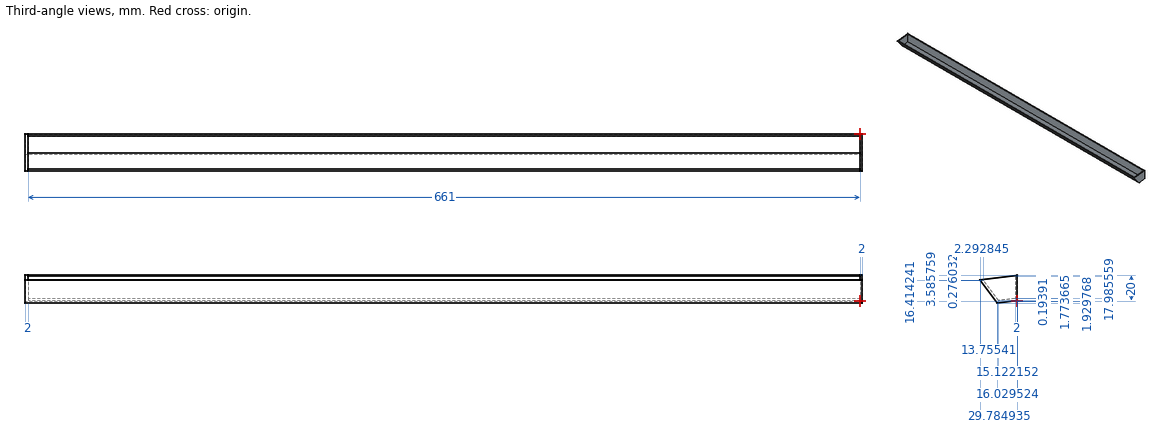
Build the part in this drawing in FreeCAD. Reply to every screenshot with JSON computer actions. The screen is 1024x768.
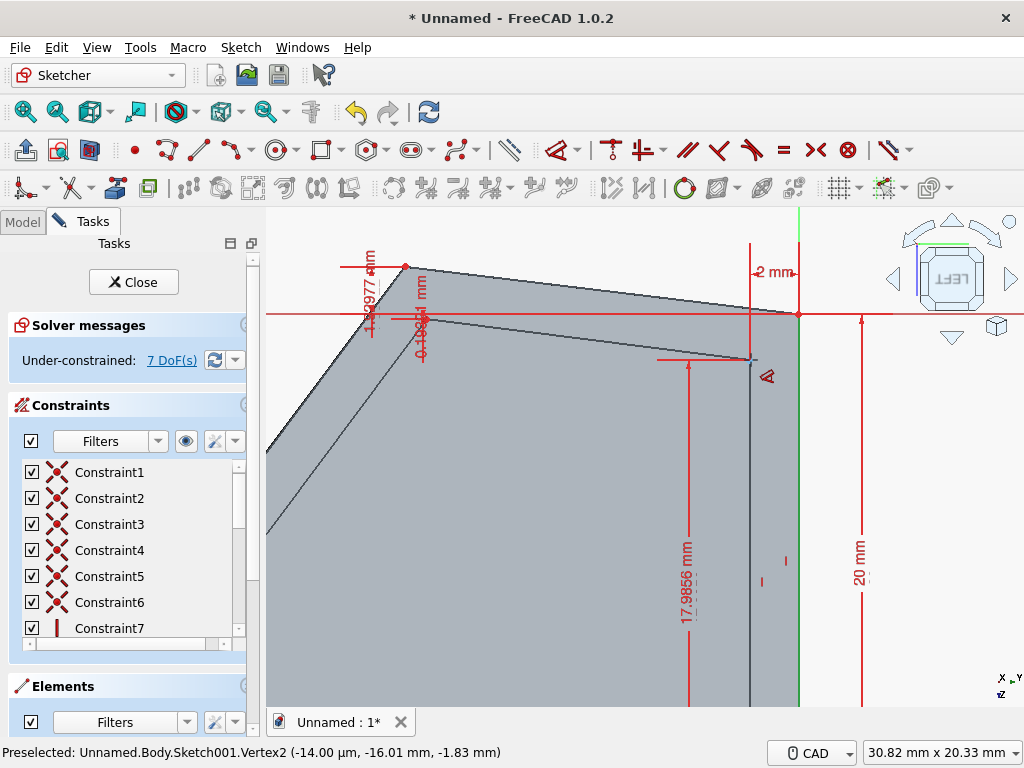
{"action": "left_click", "coordinate": [750, 360]}
{"action": "left_click", "coordinate": [833, 337]}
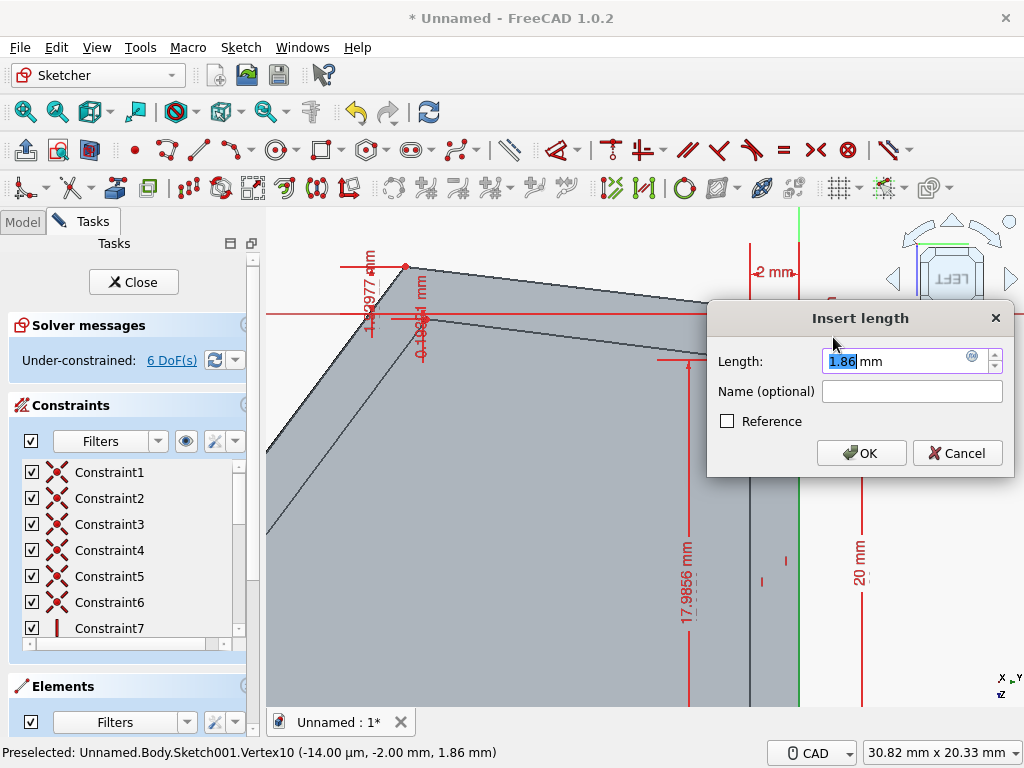
{"action": "type", "text": "1.773665"}
{"action": "key", "text": "Return"}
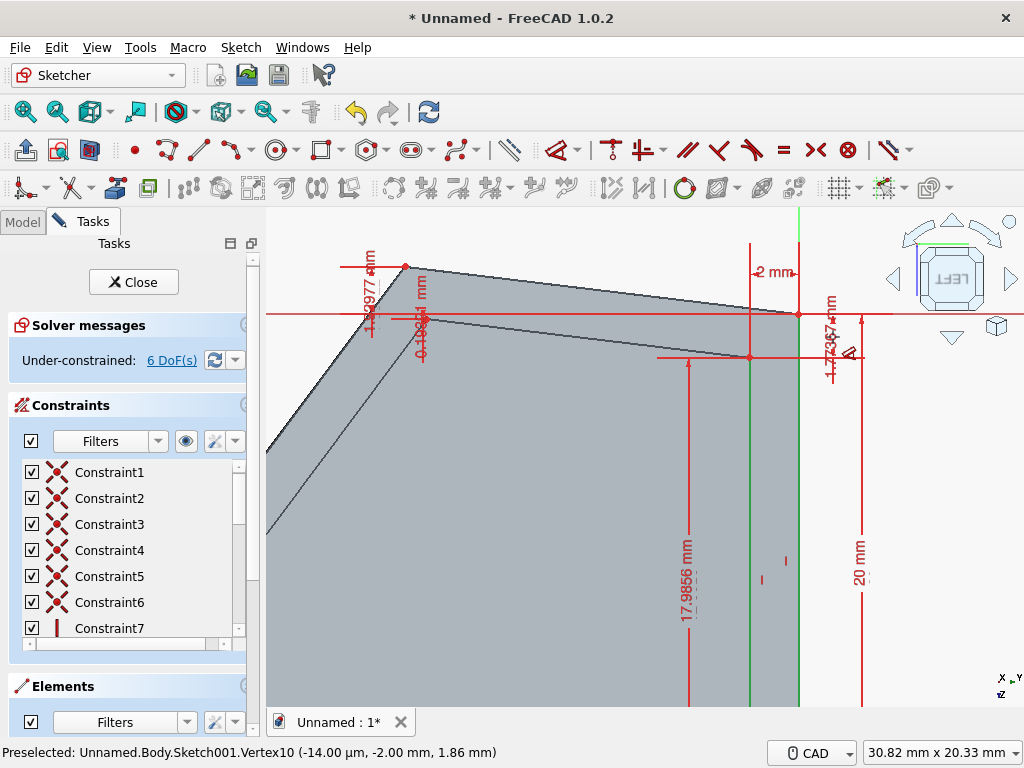
{"action": "left_click", "coordinate": [304, 403]}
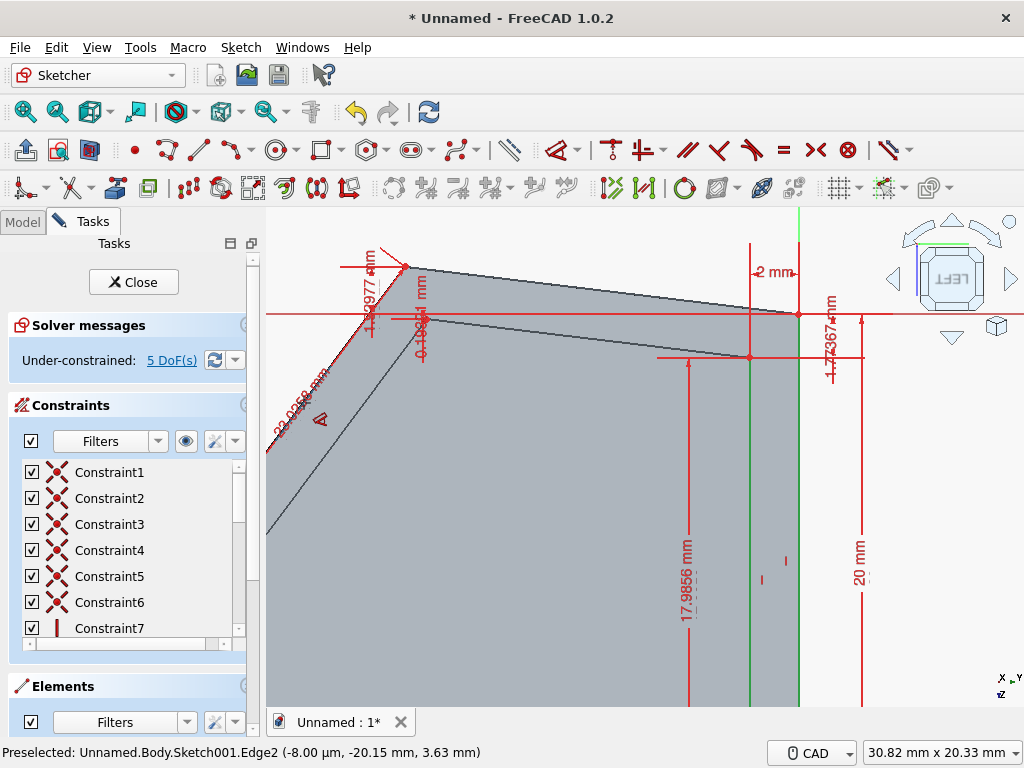
{"action": "key", "text": "Escape"}
{"action": "key", "text": "Escape"}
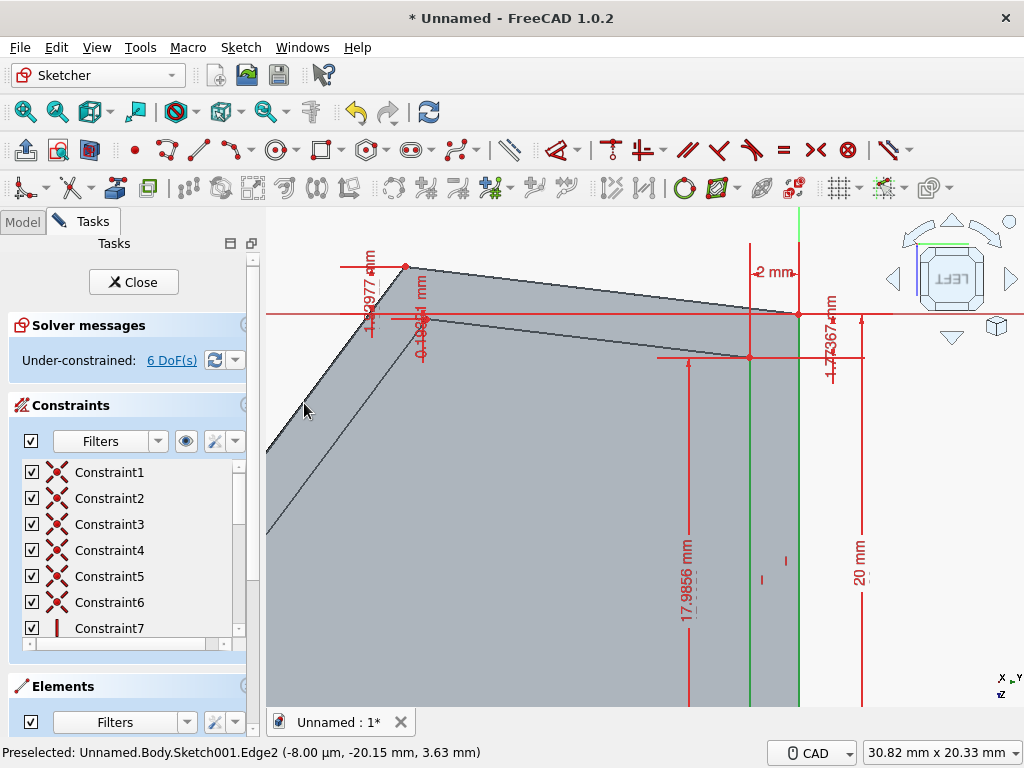
{"action": "left_click", "coordinate": [304, 403]}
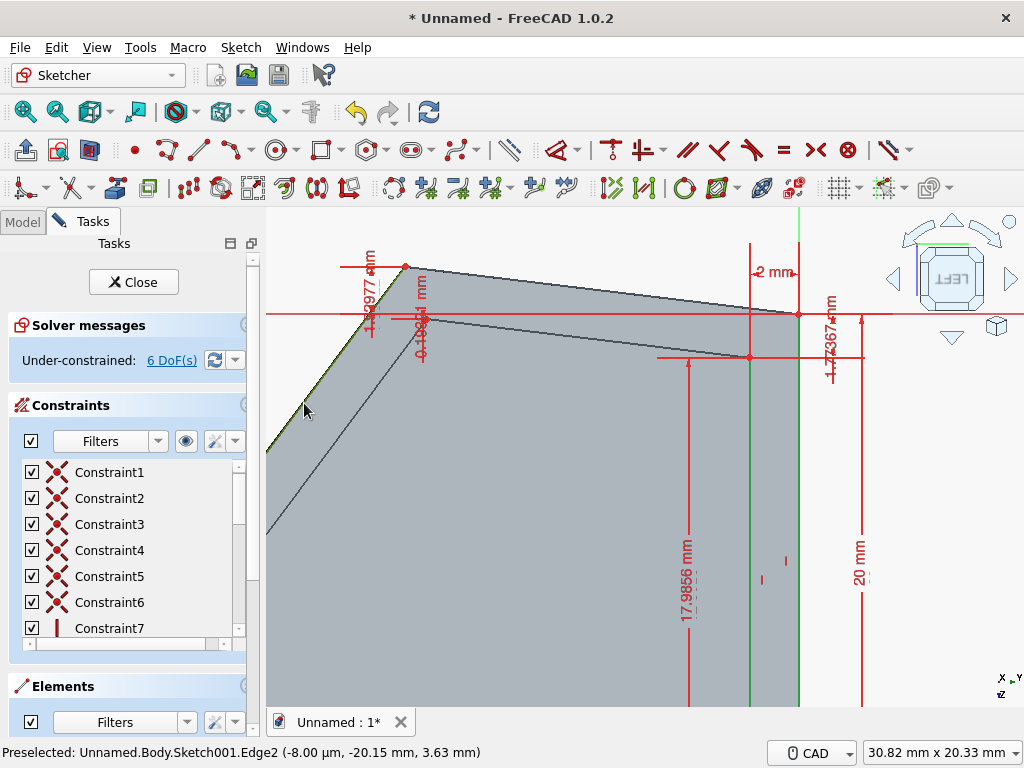
{"action": "key", "text": "l"}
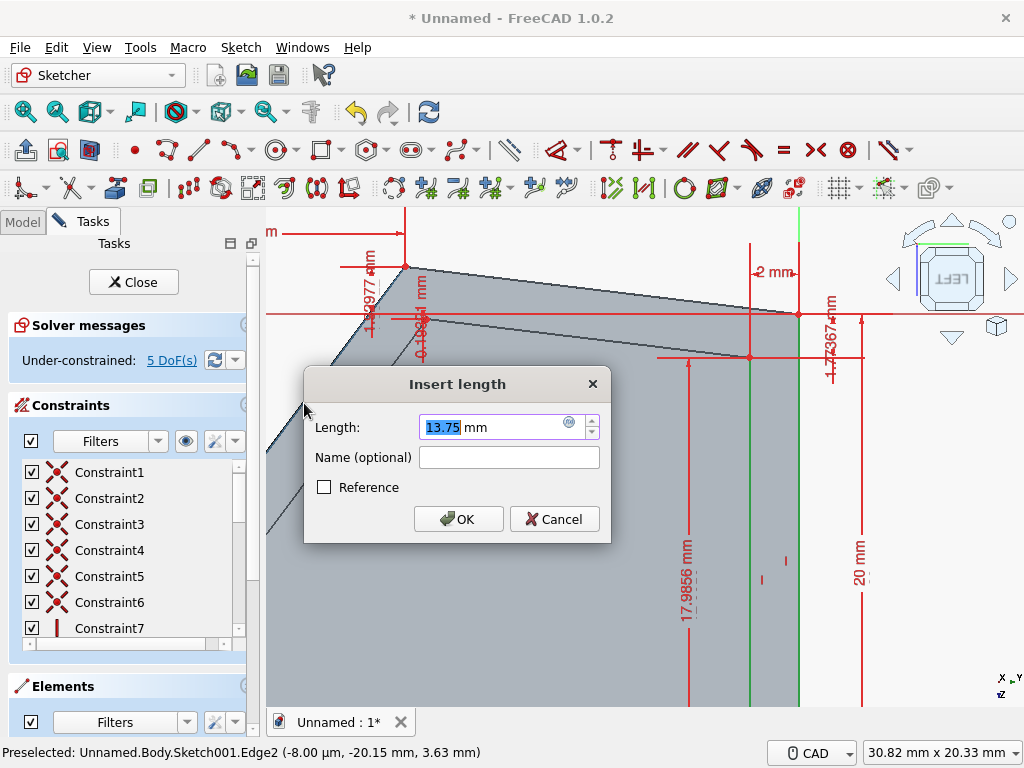
{"action": "type", "text": "13.75541"}
{"action": "key", "text": "Return"}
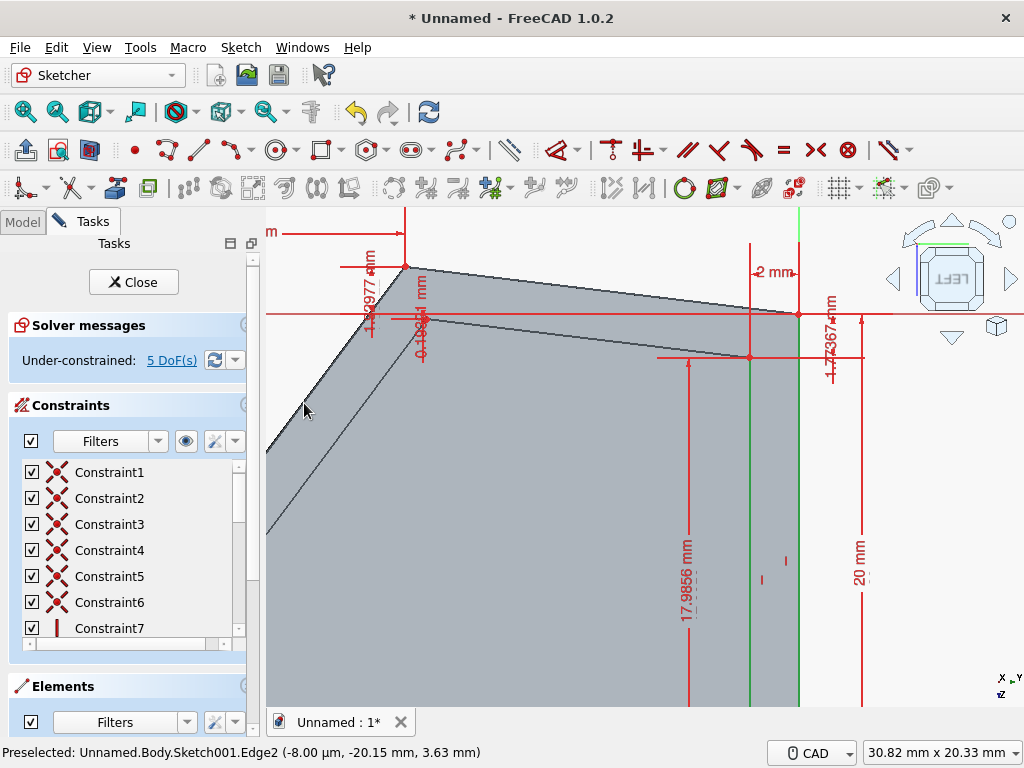
{"action": "scroll", "coordinate": [751, 360], "scroll_direction": "down", "scroll_amount": 3}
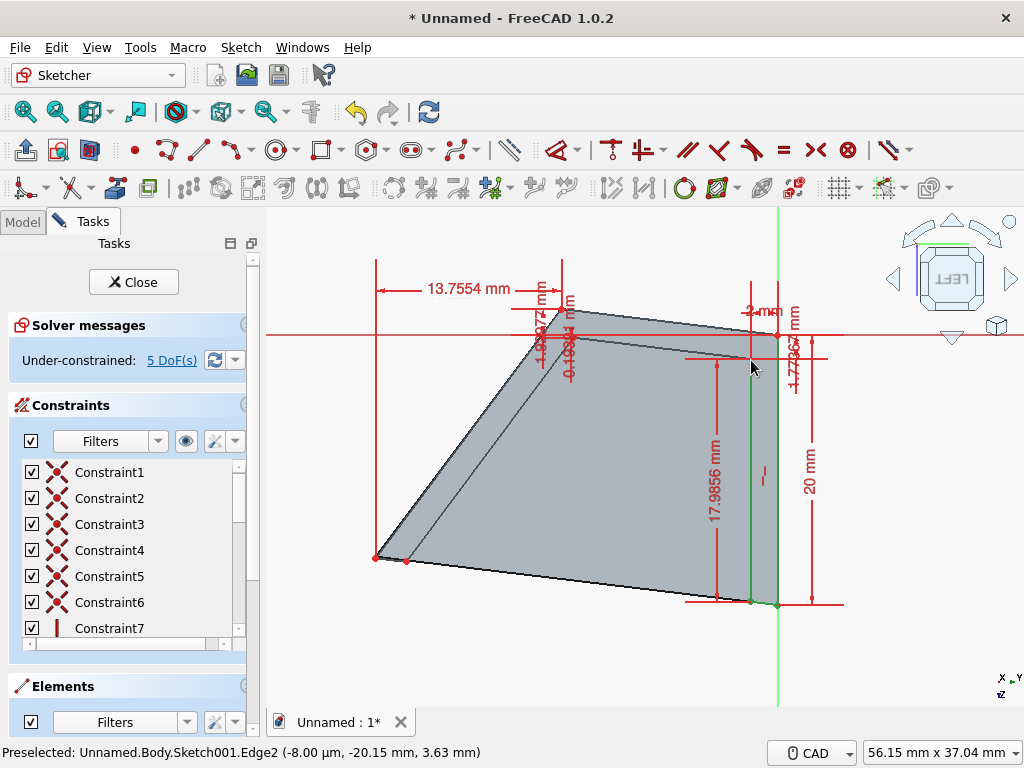
{"action": "scroll", "coordinate": [385, 559], "scroll_direction": "up", "scroll_amount": 3}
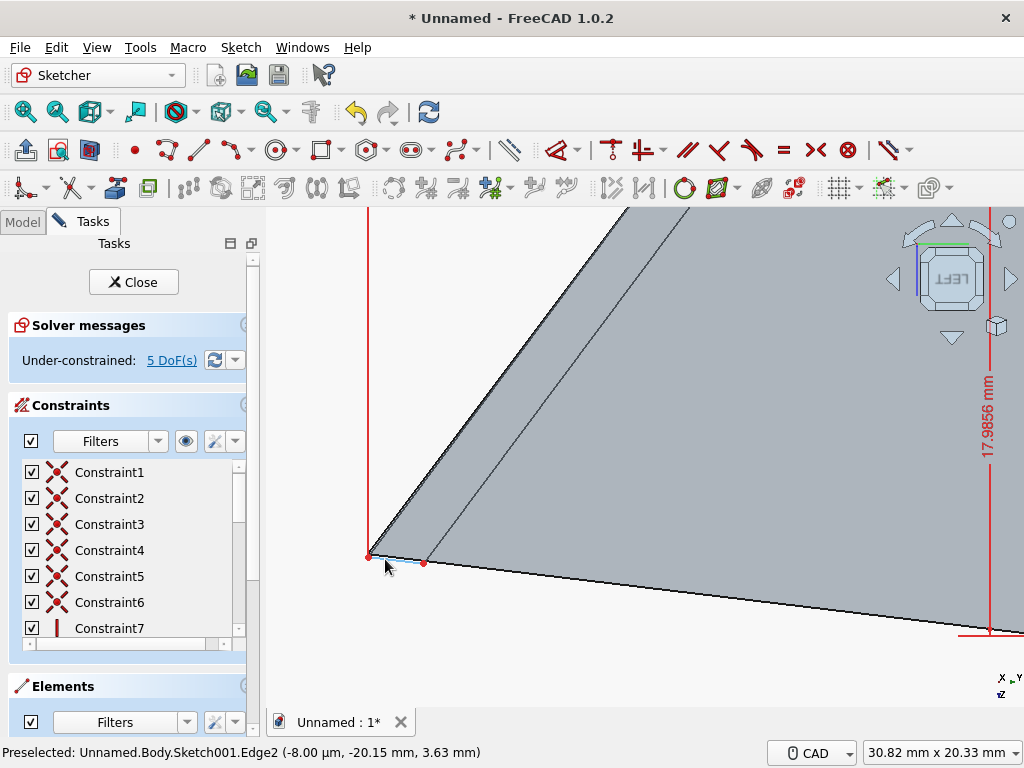
{"action": "left_click", "coordinate": [385, 559]}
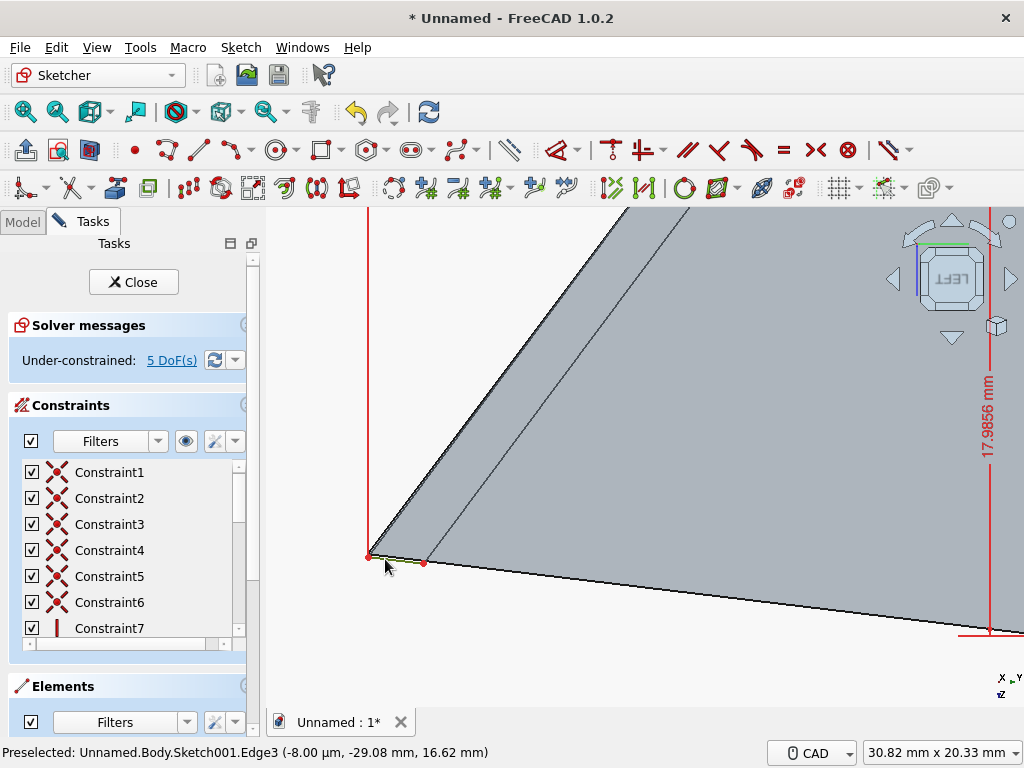
{"action": "key", "text": "l"}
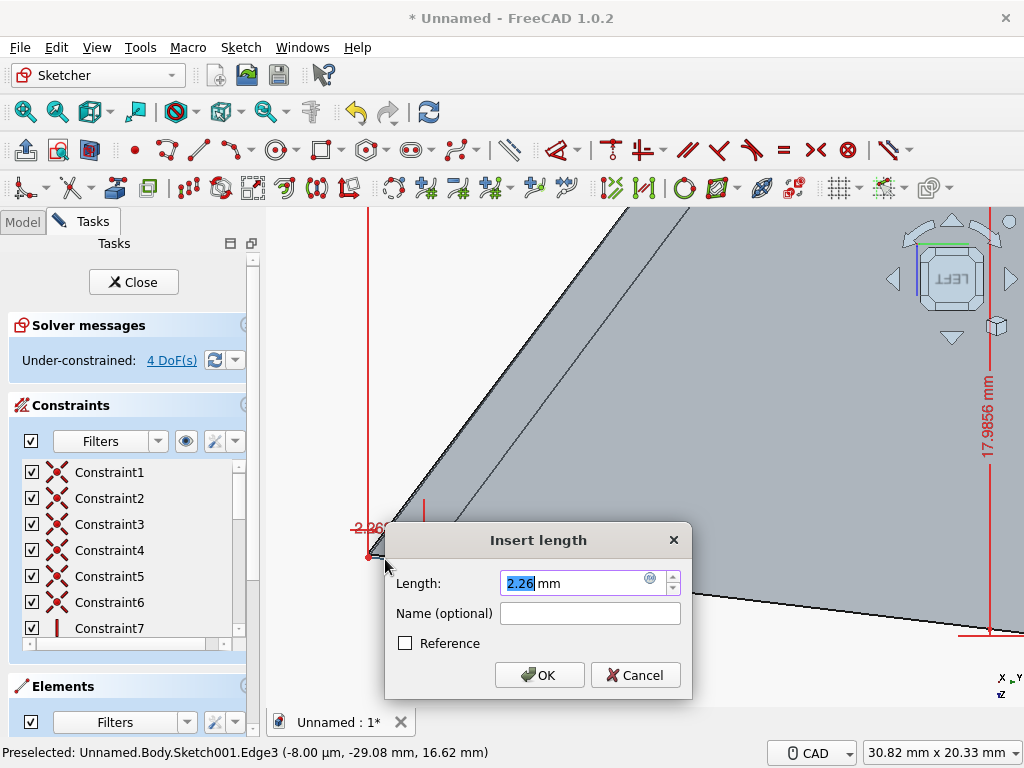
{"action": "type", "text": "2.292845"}
{"action": "key", "text": "Return"}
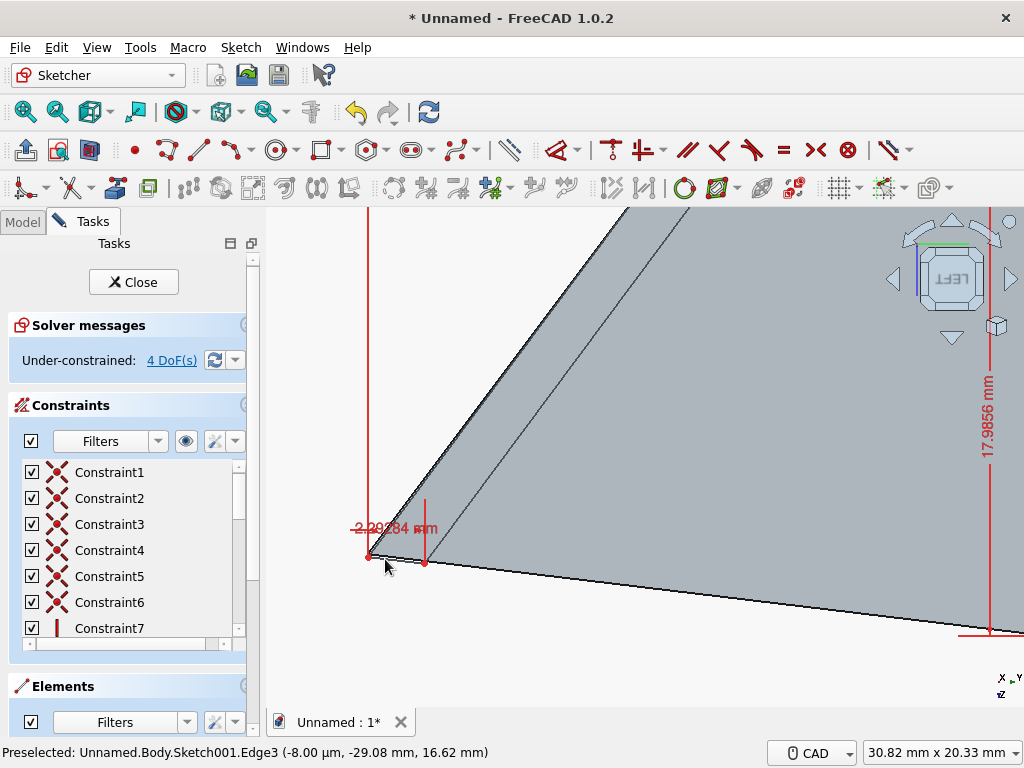
{"action": "scroll", "coordinate": [385, 559], "scroll_direction": "up", "scroll_amount": 9}